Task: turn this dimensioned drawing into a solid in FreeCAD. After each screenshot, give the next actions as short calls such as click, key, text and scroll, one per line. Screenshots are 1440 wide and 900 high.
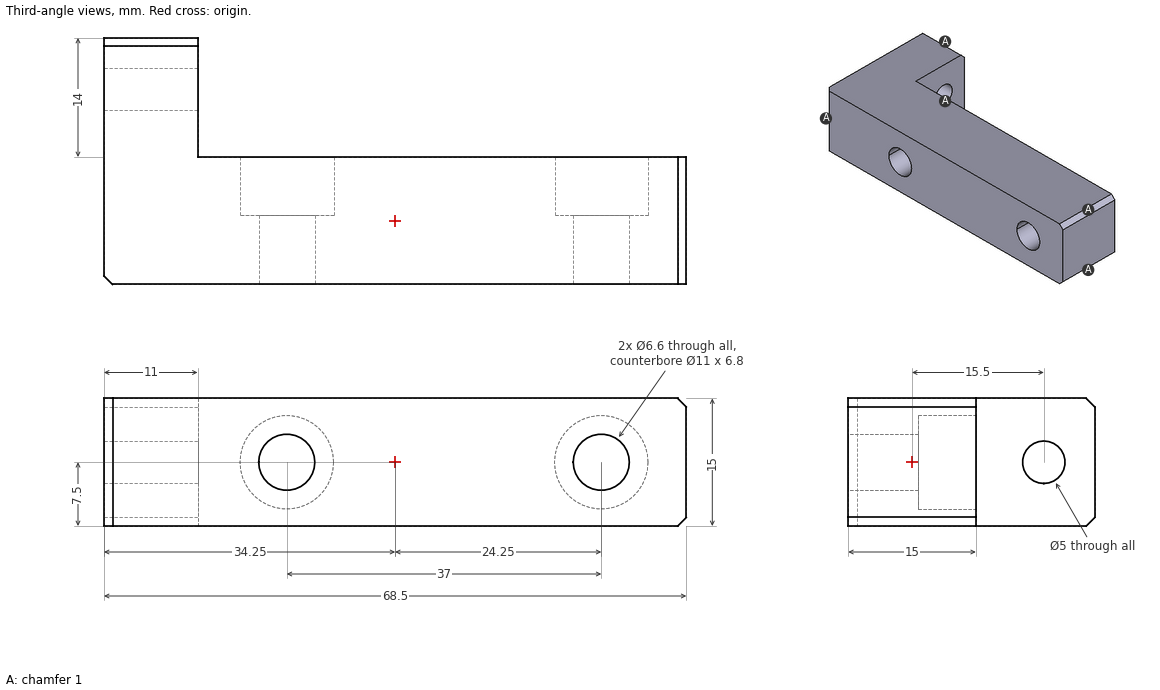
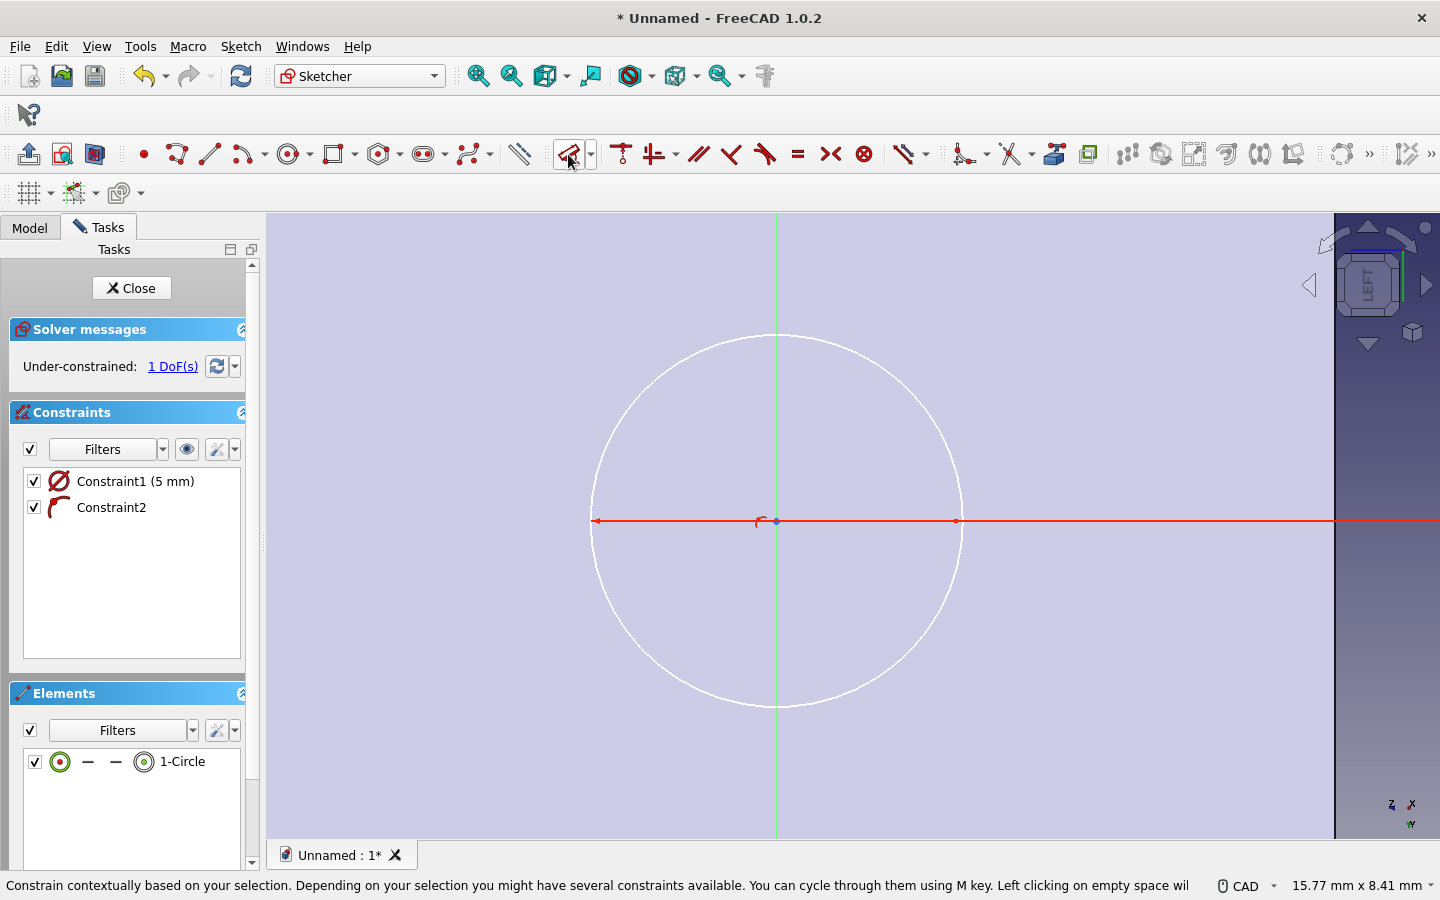
click(777, 521)
click(811, 381)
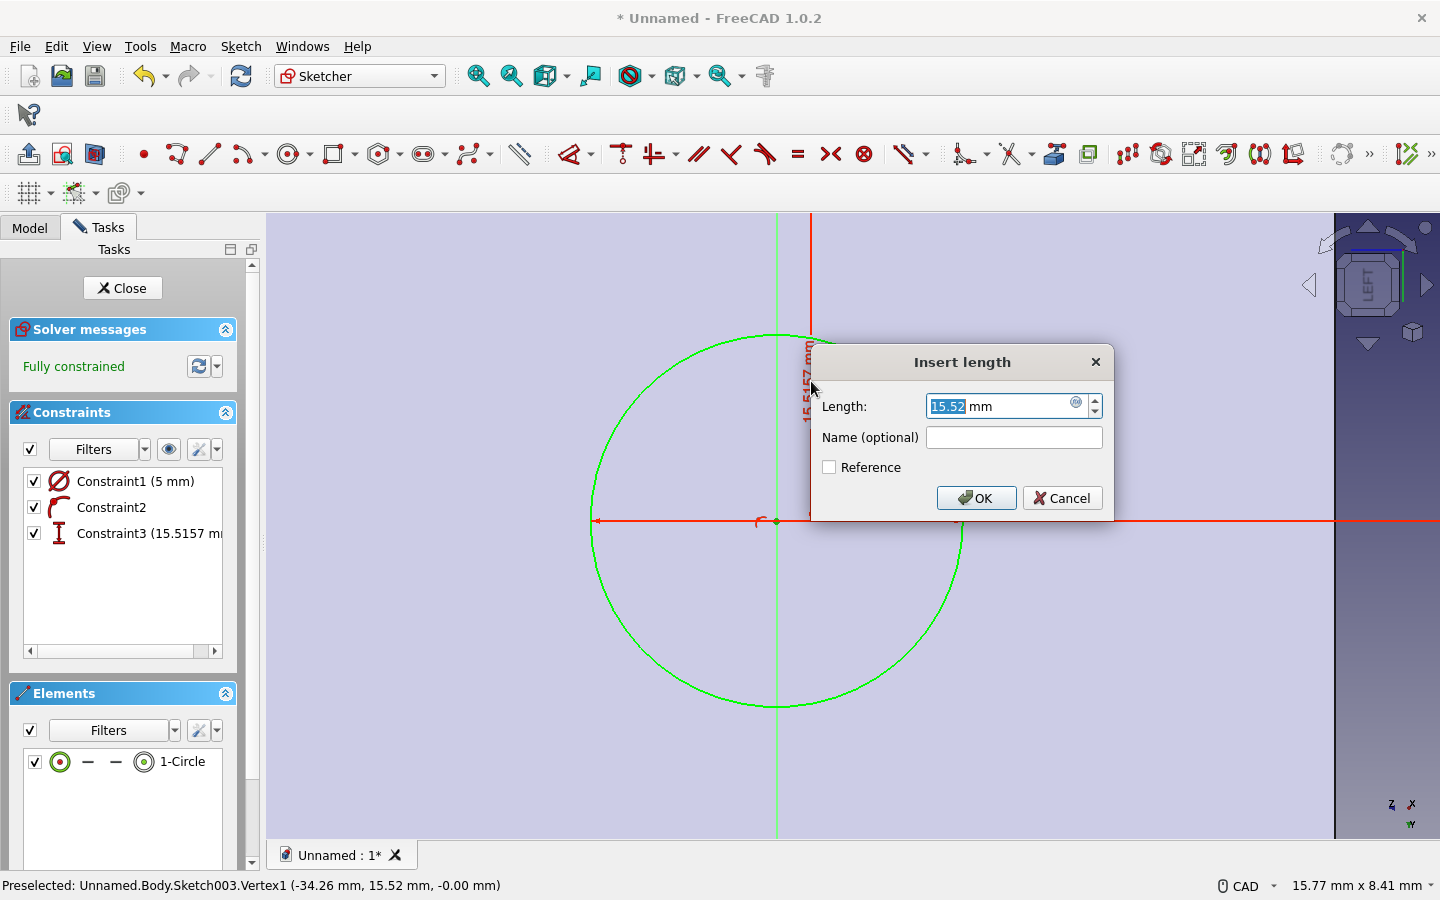
text(15.5)
key(Return)
key(Escape)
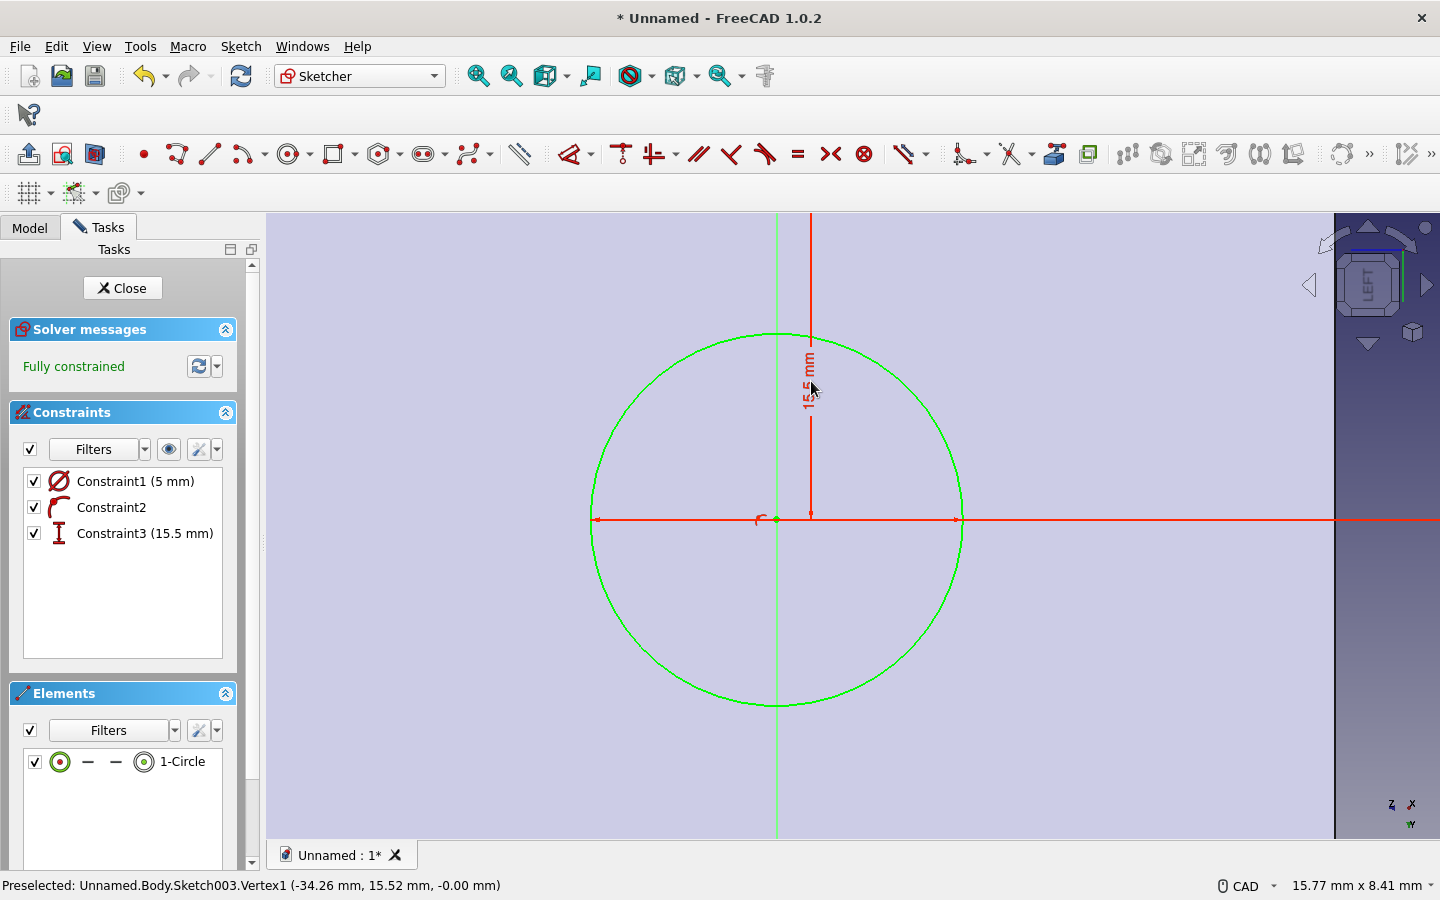
click(123, 288)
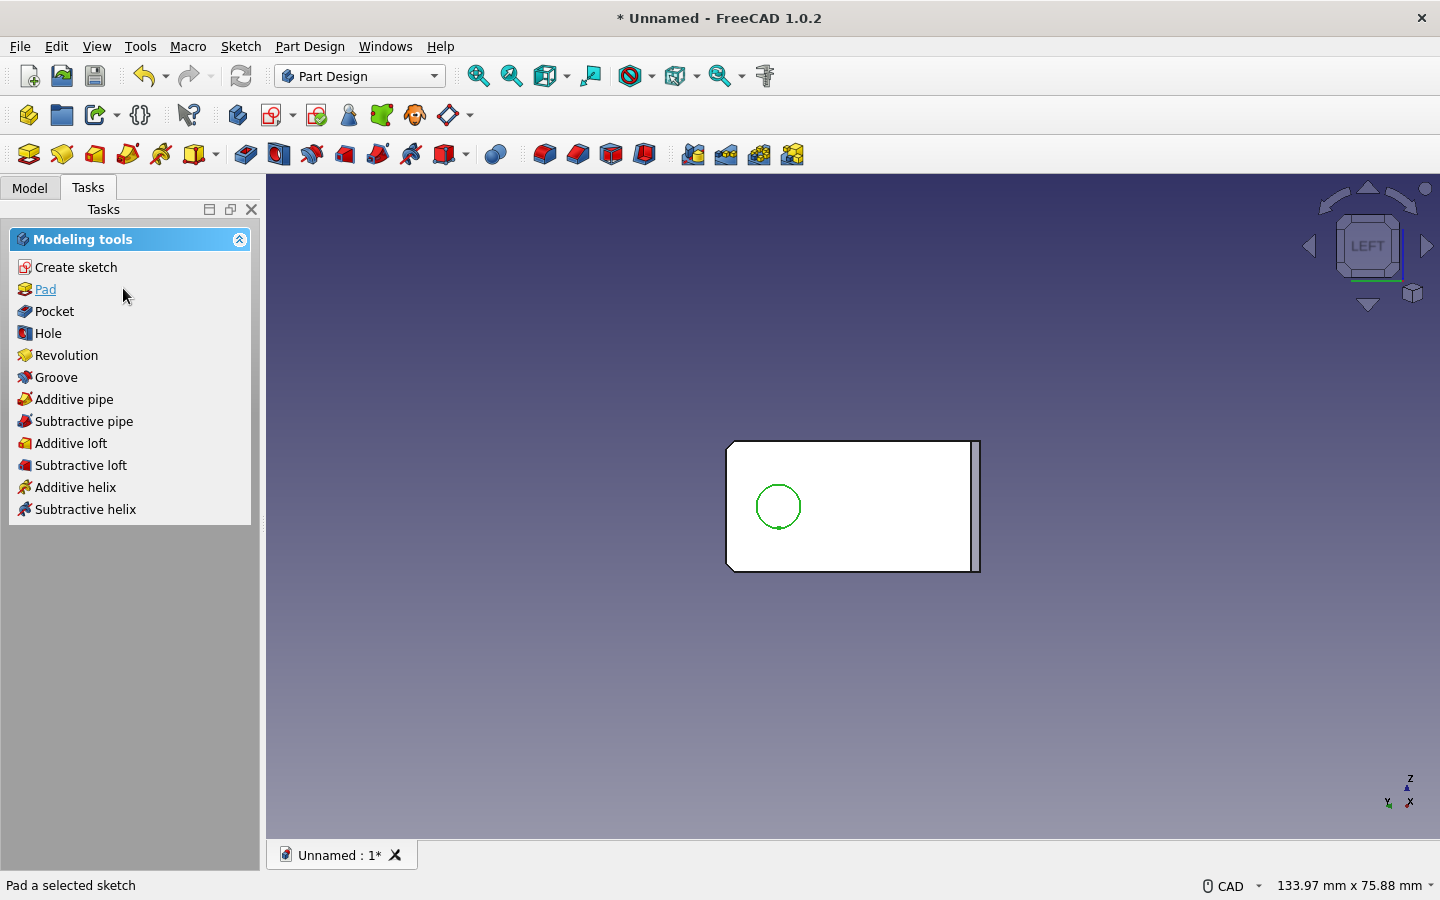
click(279, 154)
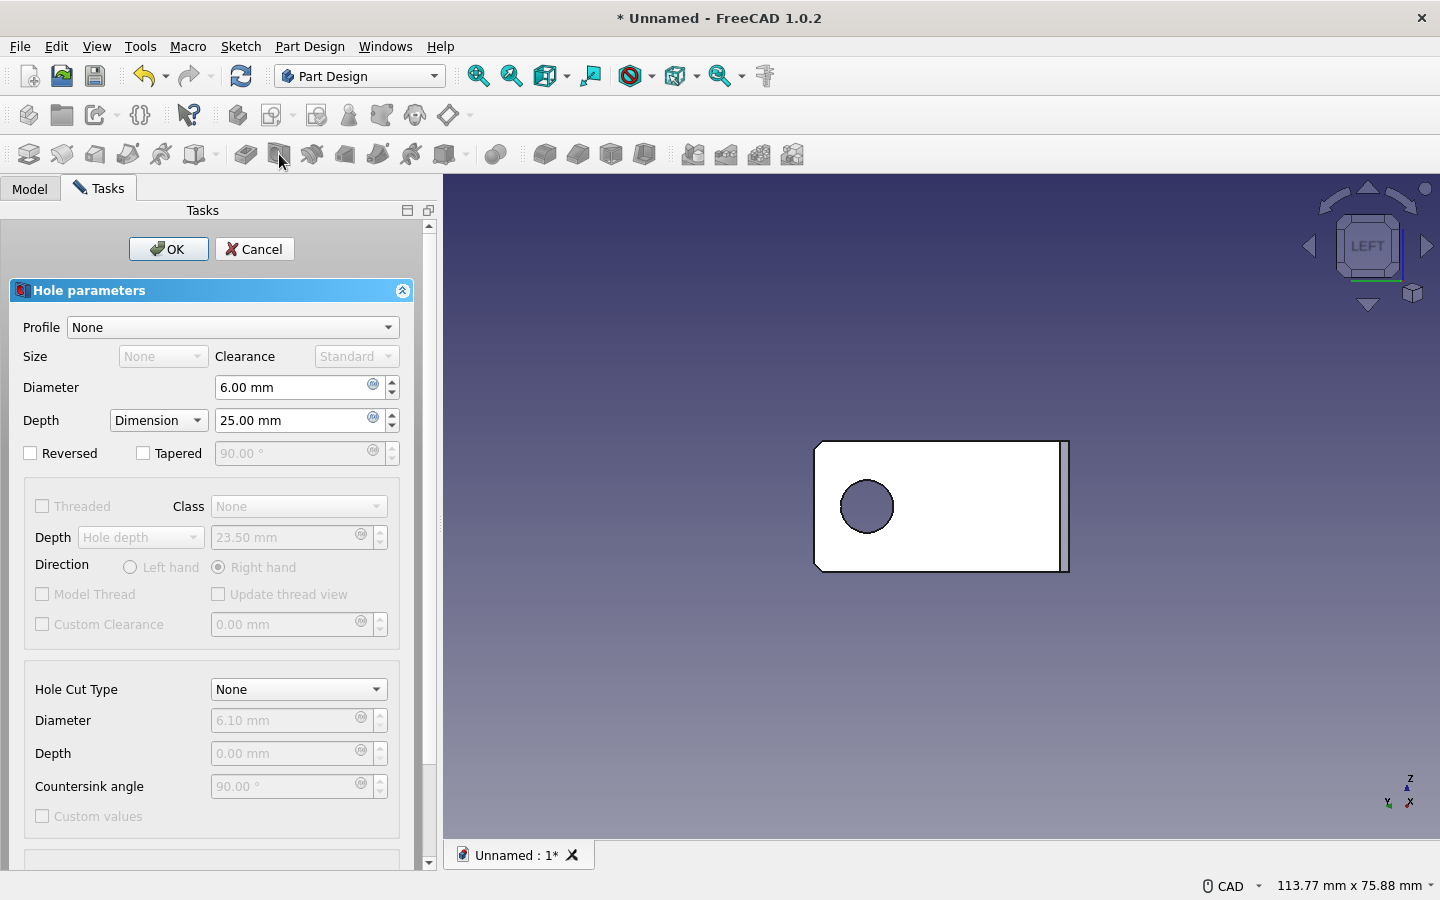
triple_click(300, 388)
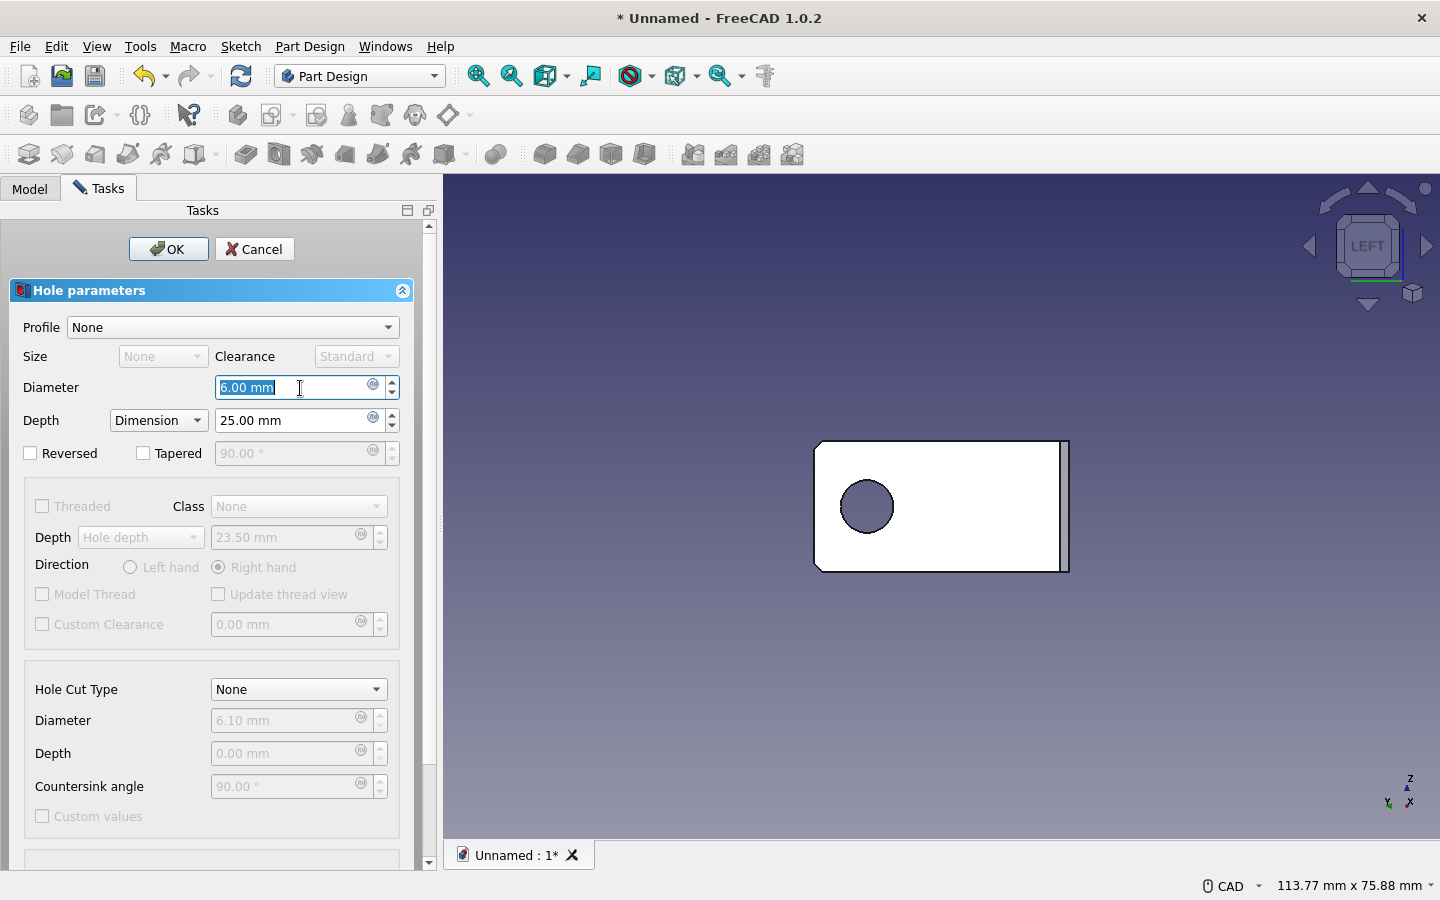
text(5)
key(Tab)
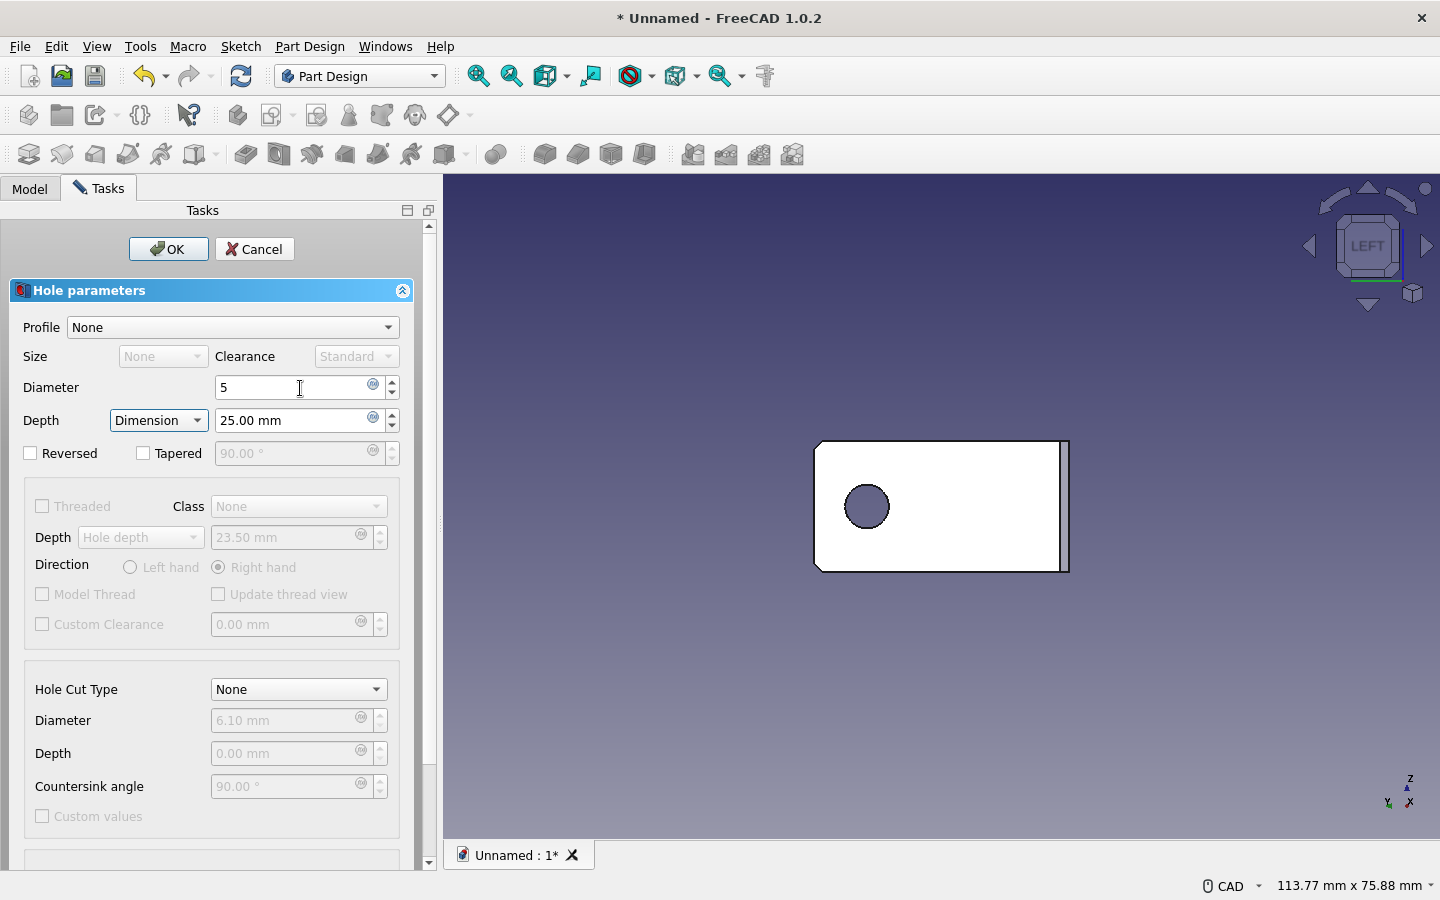
click(160, 420)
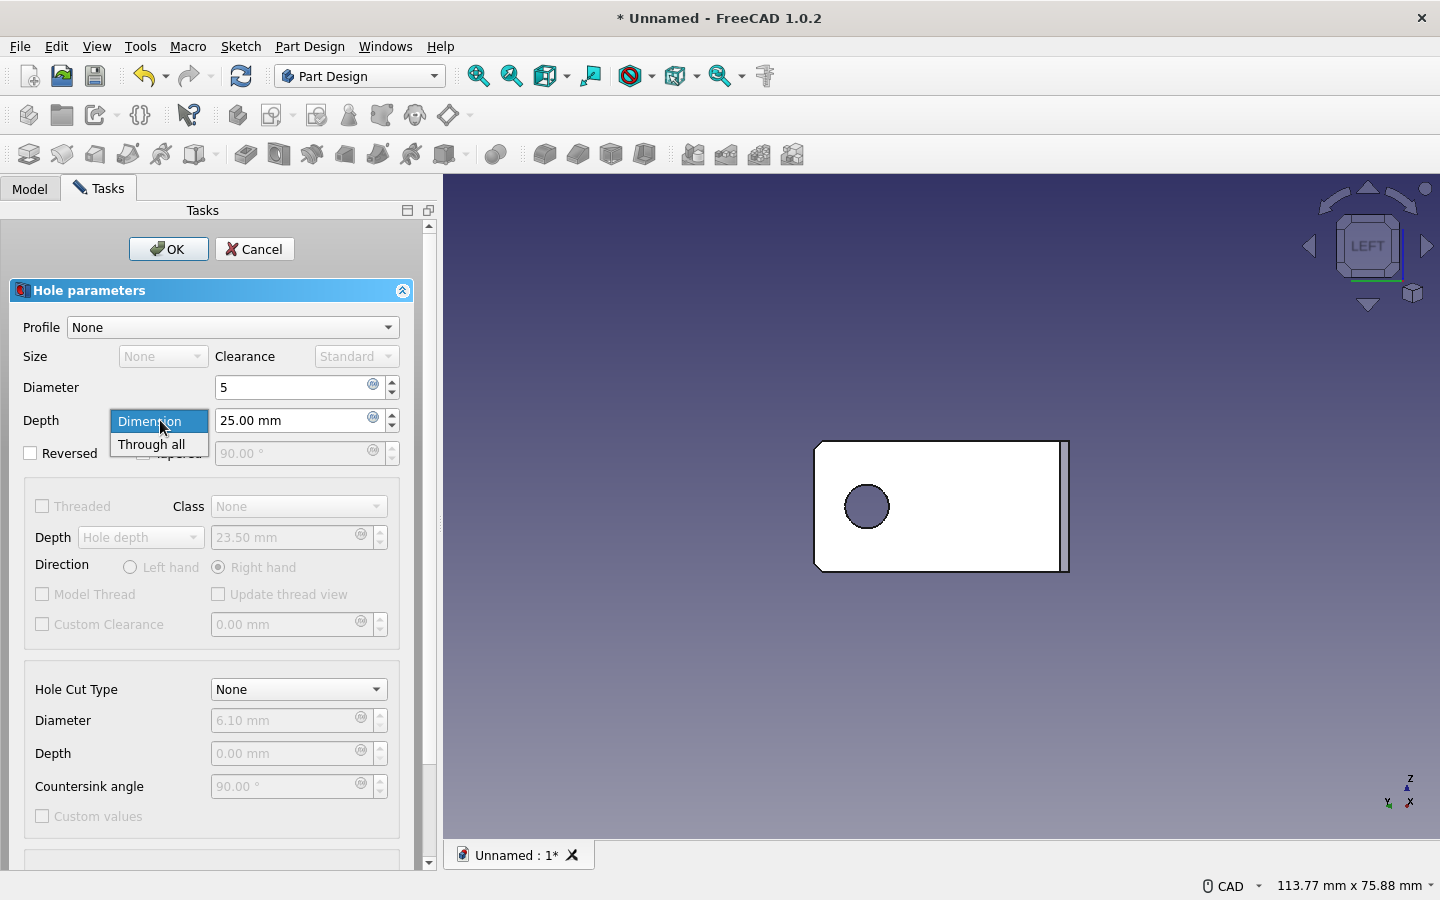
click(158, 444)